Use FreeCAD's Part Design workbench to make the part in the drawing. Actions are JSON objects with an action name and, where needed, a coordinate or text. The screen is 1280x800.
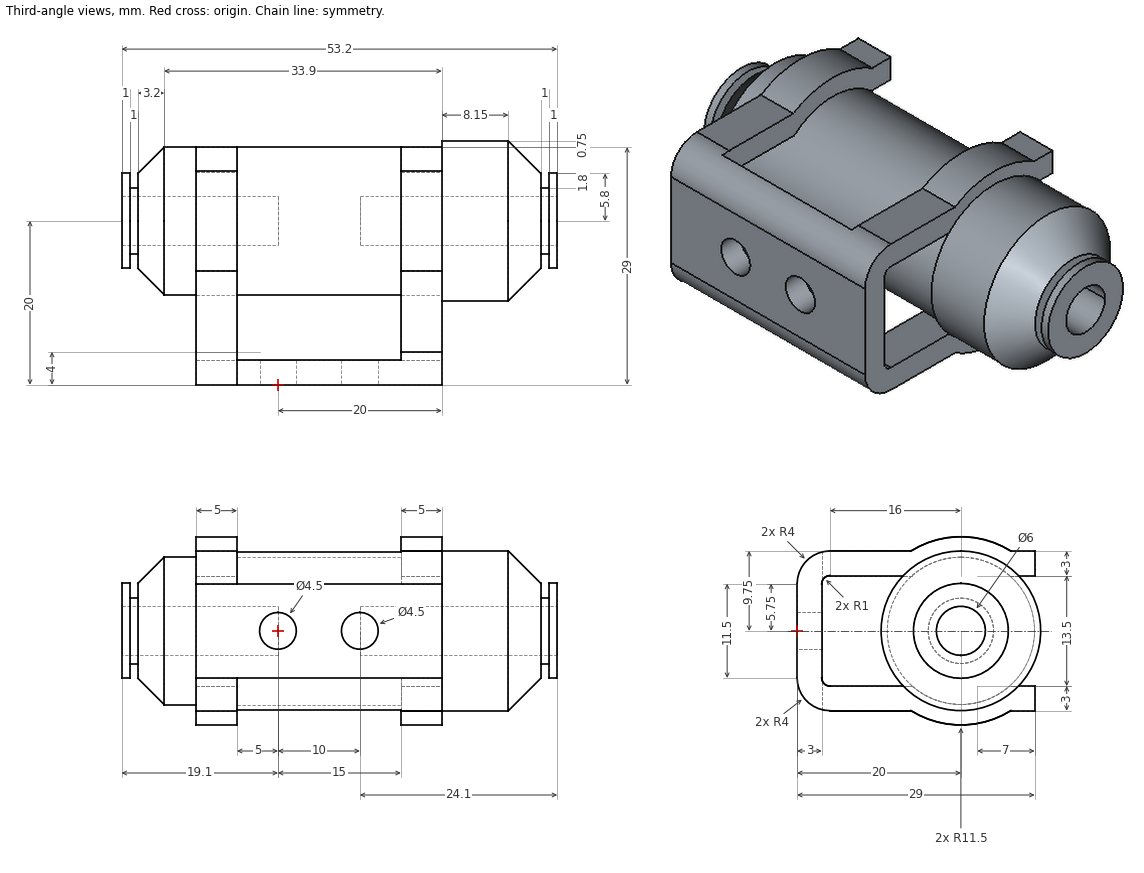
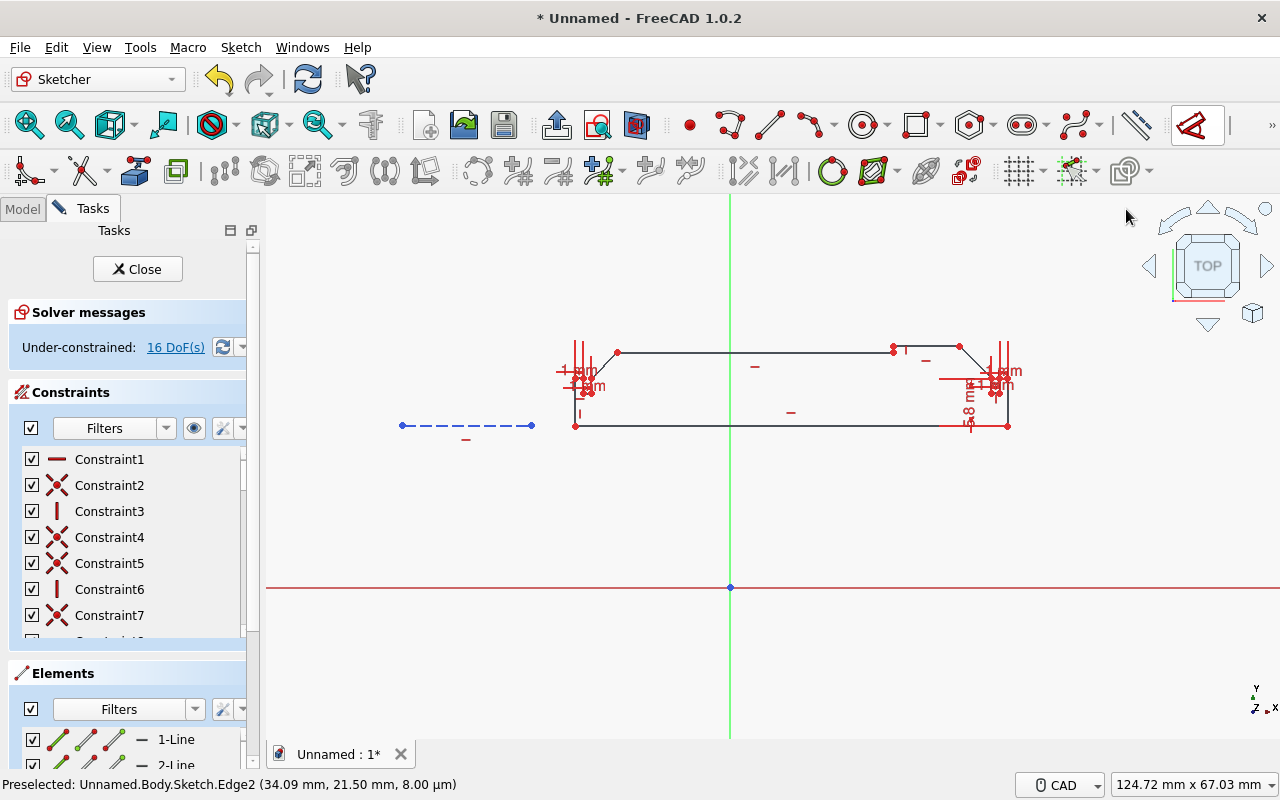
{"action": "scroll", "coordinate": [1000, 386], "scroll_direction": "up", "scroll_amount": 5}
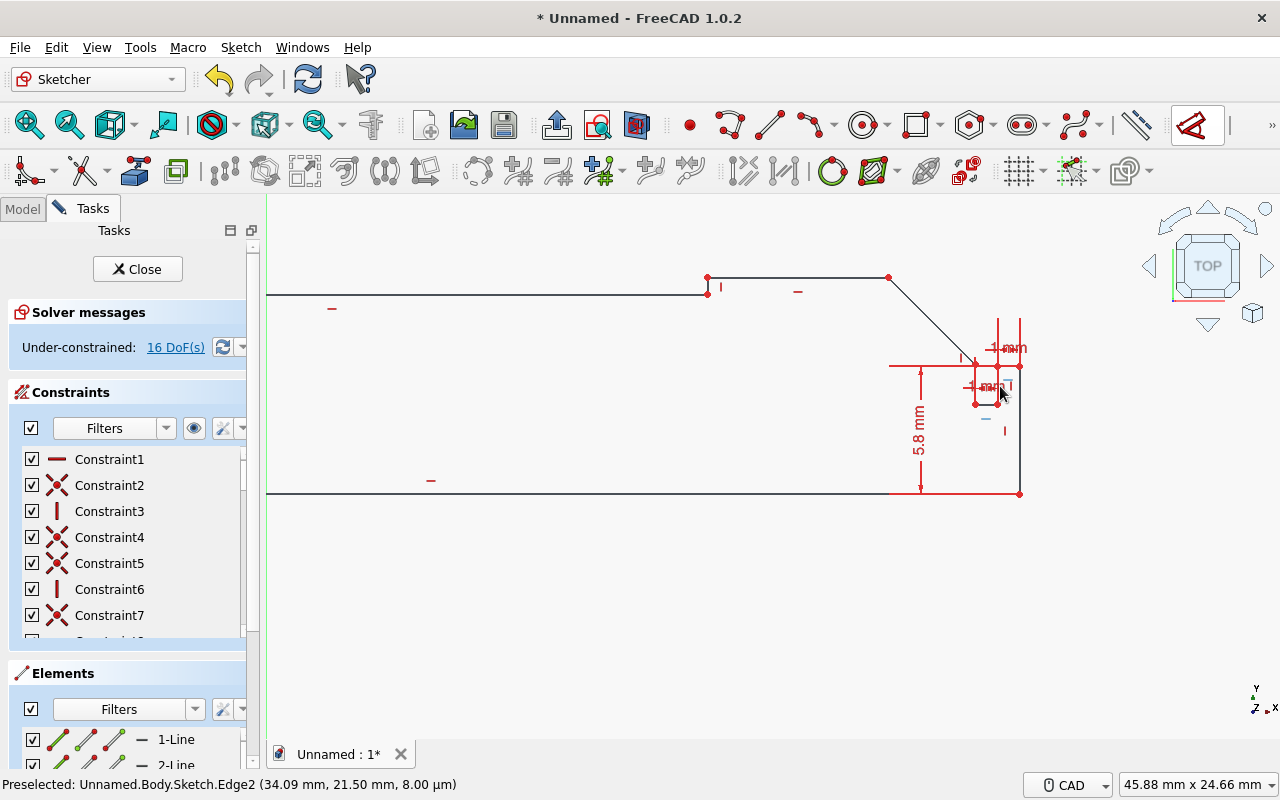
{"action": "left_click", "coordinate": [998, 378]}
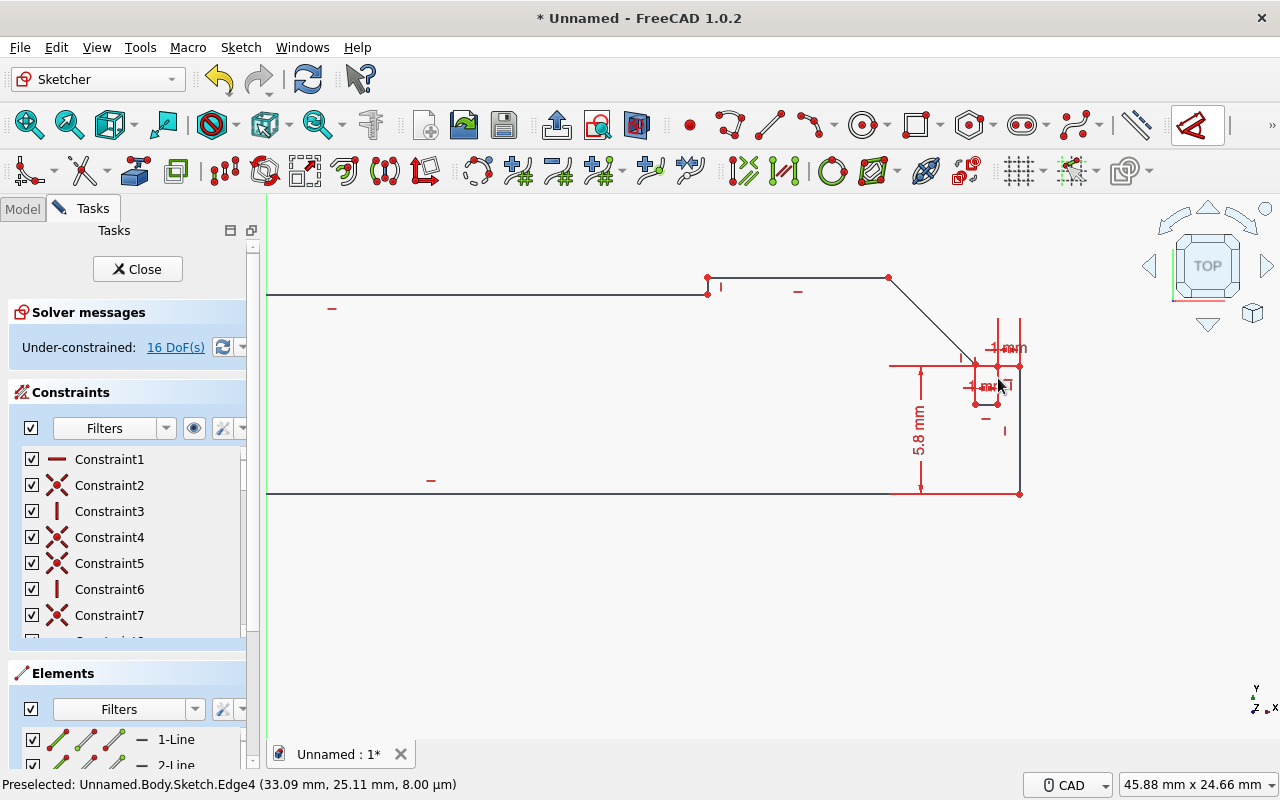
{"action": "left_click", "coordinate": [1218, 126]}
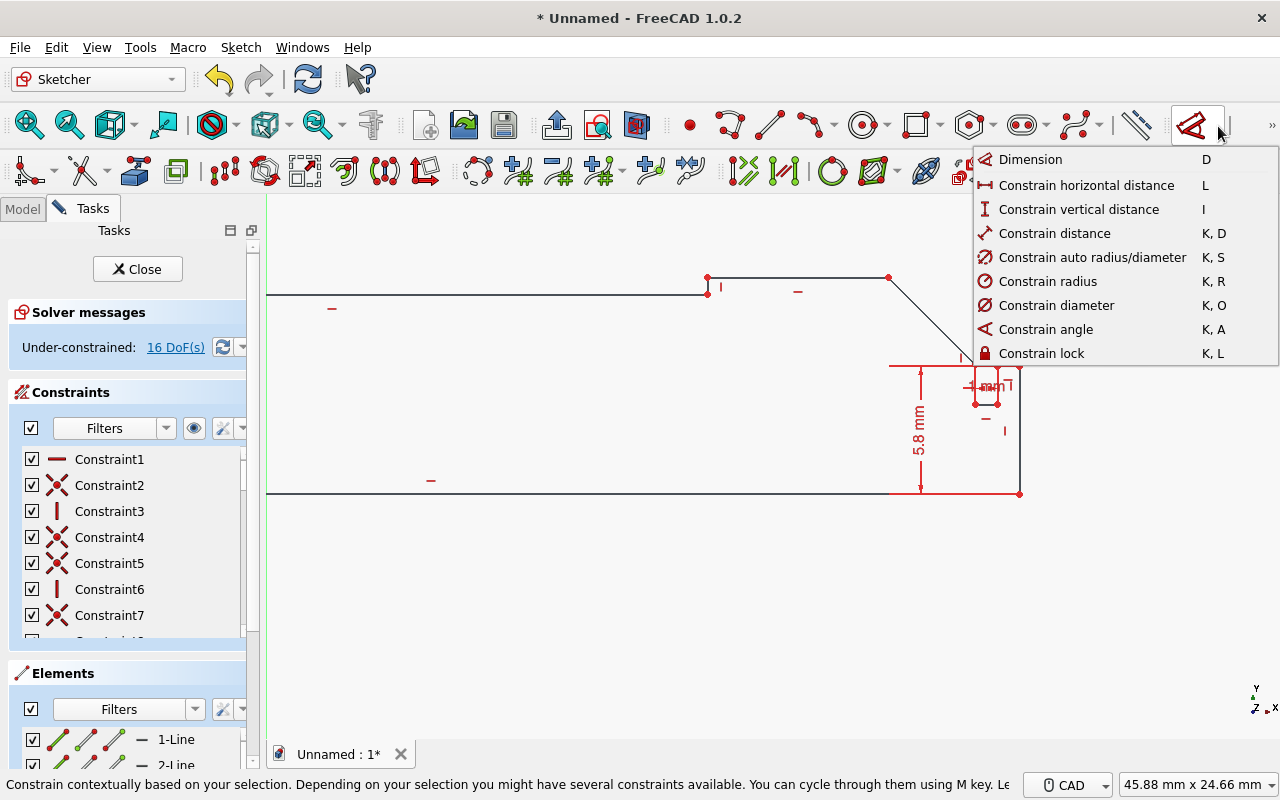
{"action": "left_click", "coordinate": [1126, 209]}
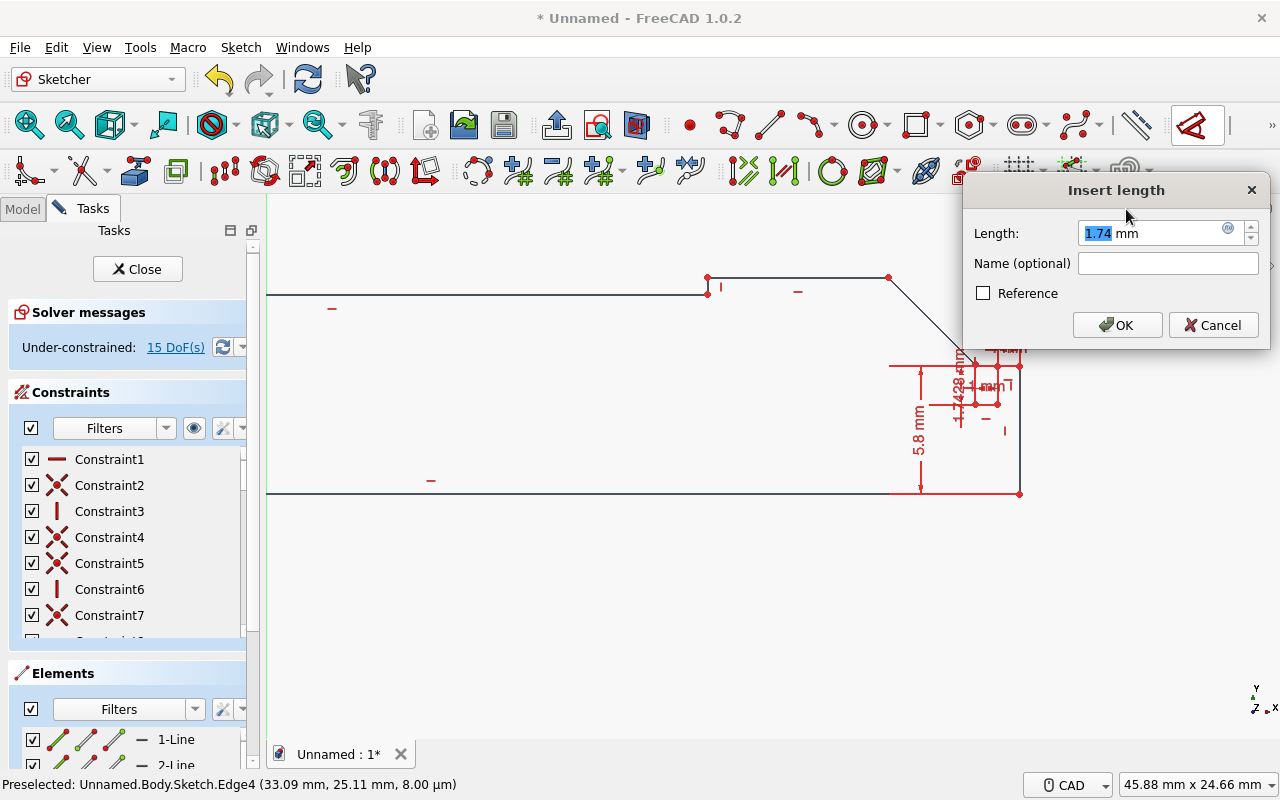
{"action": "type", "text": "1.8"}
{"action": "key", "text": "Return"}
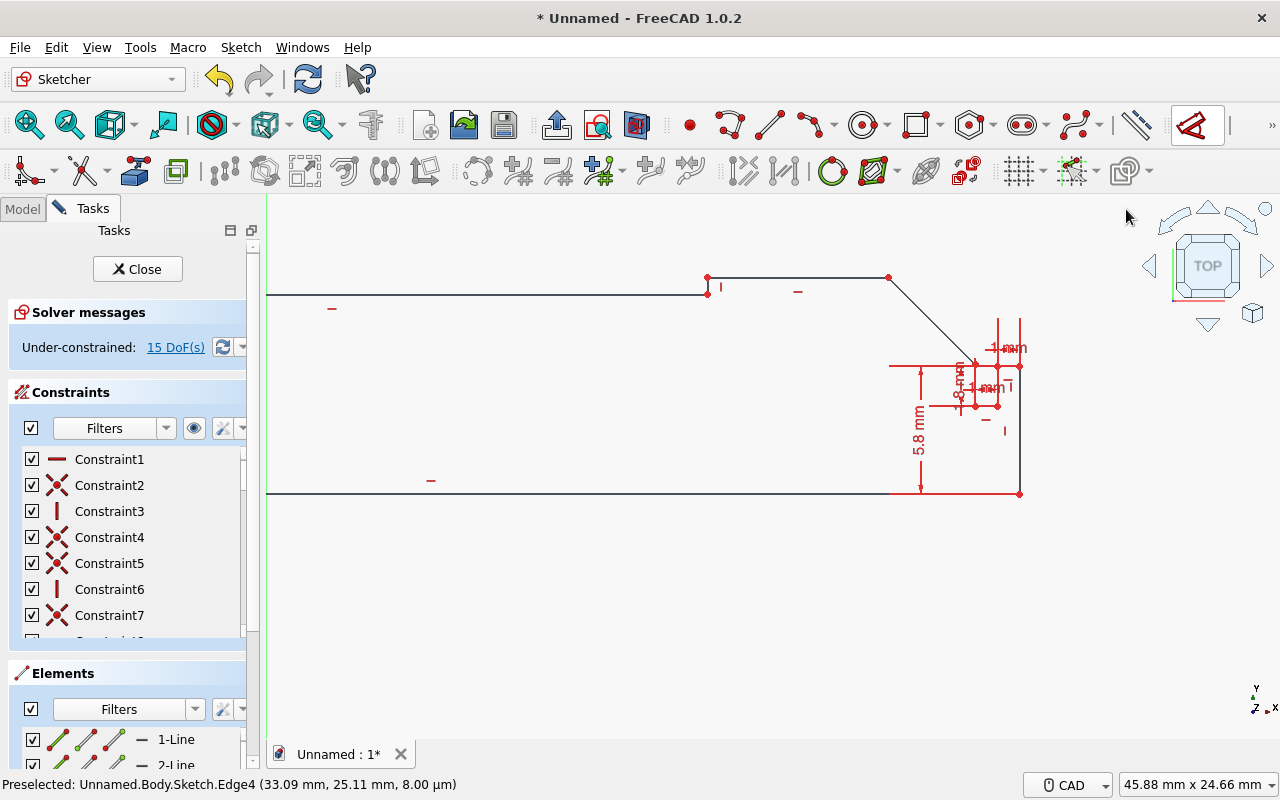
{"action": "left_click", "coordinate": [975, 377]}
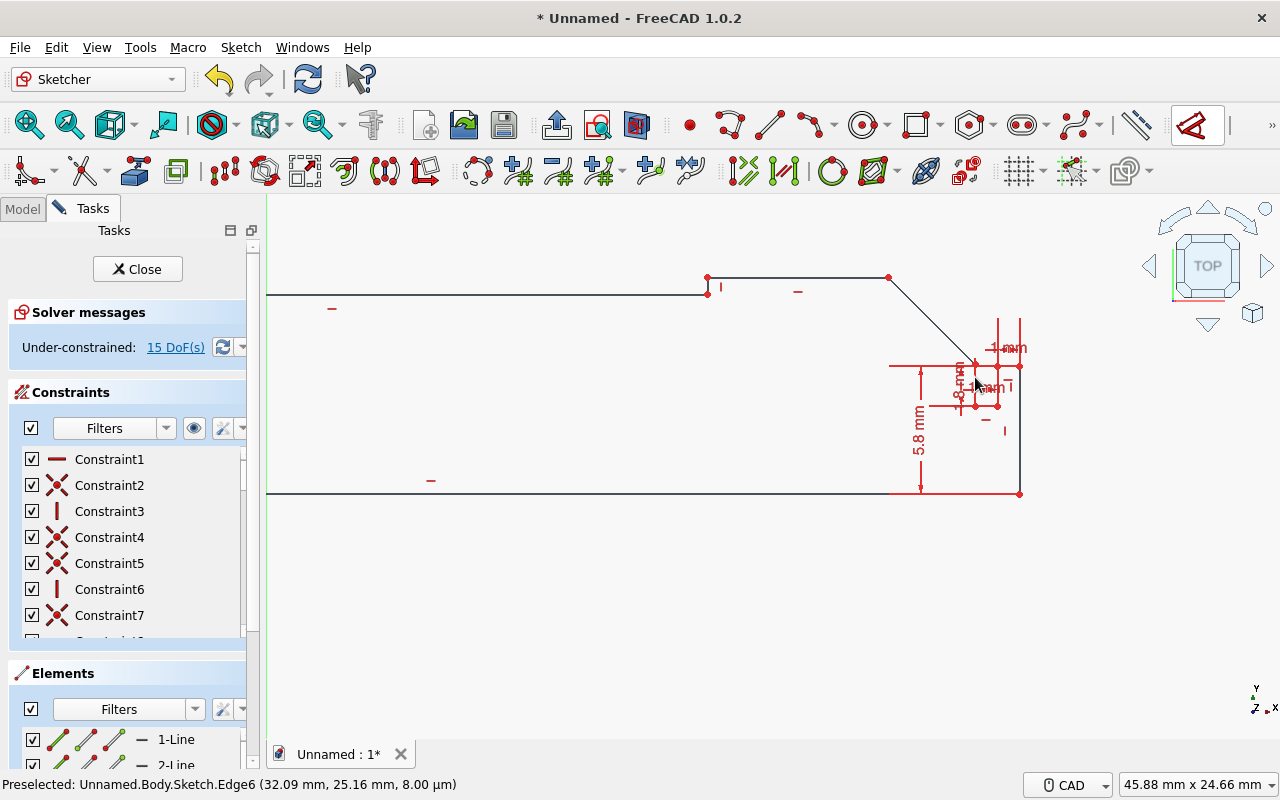
{"action": "left_click", "coordinate": [1218, 126]}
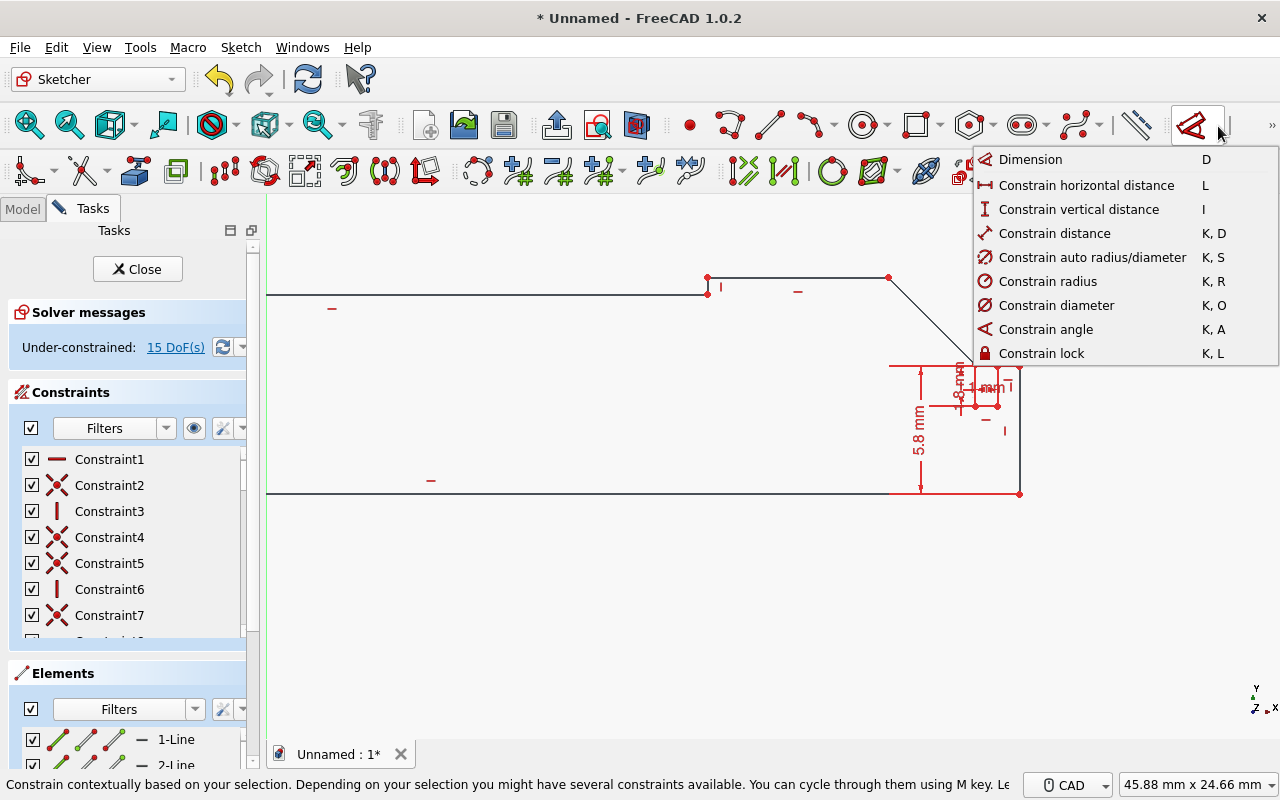
{"action": "left_click", "coordinate": [1126, 209]}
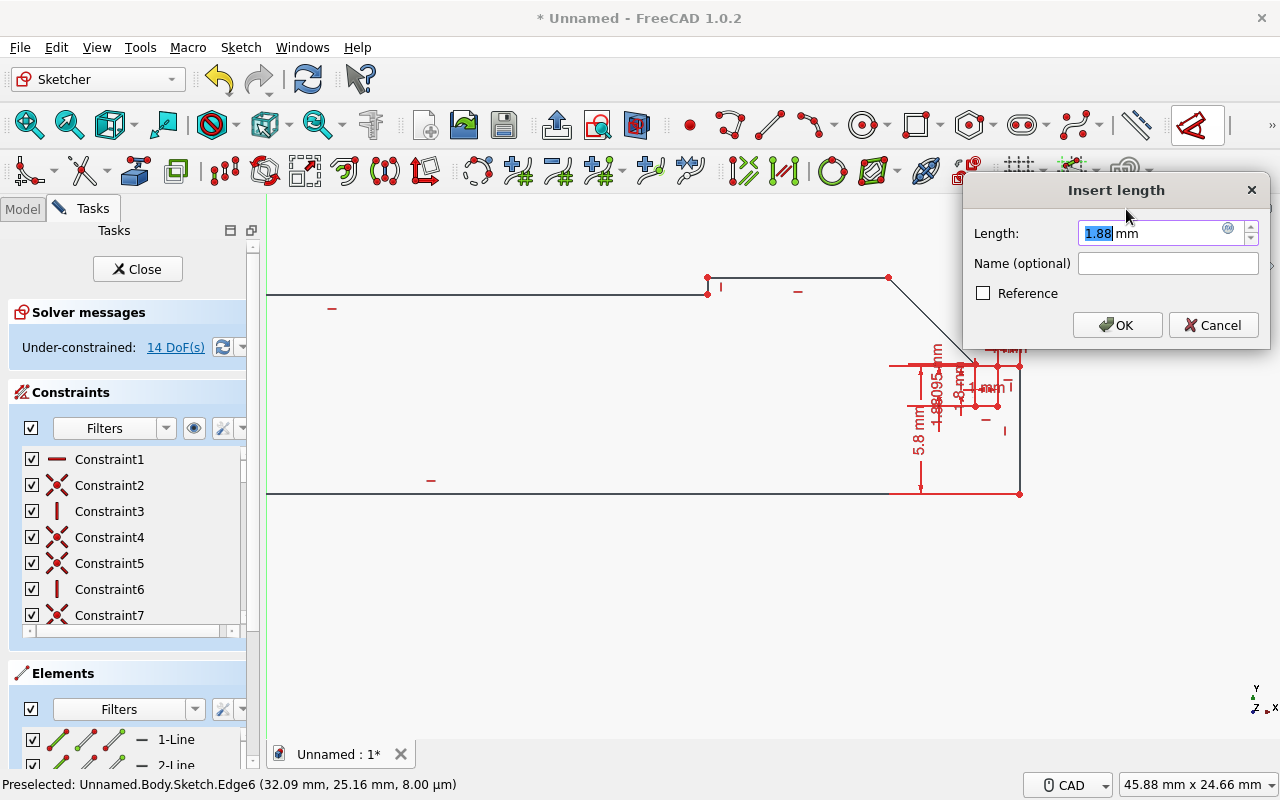
{"action": "type", "text": "1.8"}
{"action": "key", "text": "Return"}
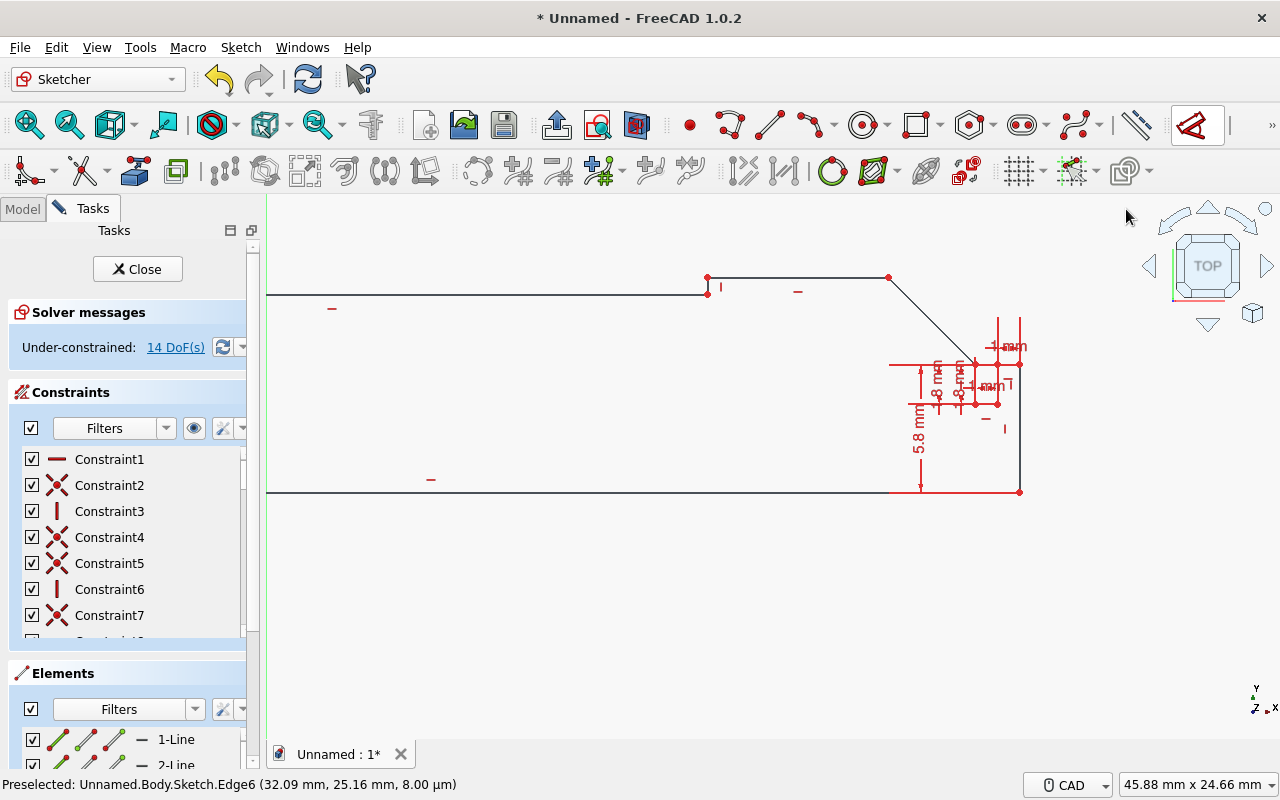
{"action": "scroll", "coordinate": [1000, 386], "scroll_direction": "down", "scroll_amount": 5}